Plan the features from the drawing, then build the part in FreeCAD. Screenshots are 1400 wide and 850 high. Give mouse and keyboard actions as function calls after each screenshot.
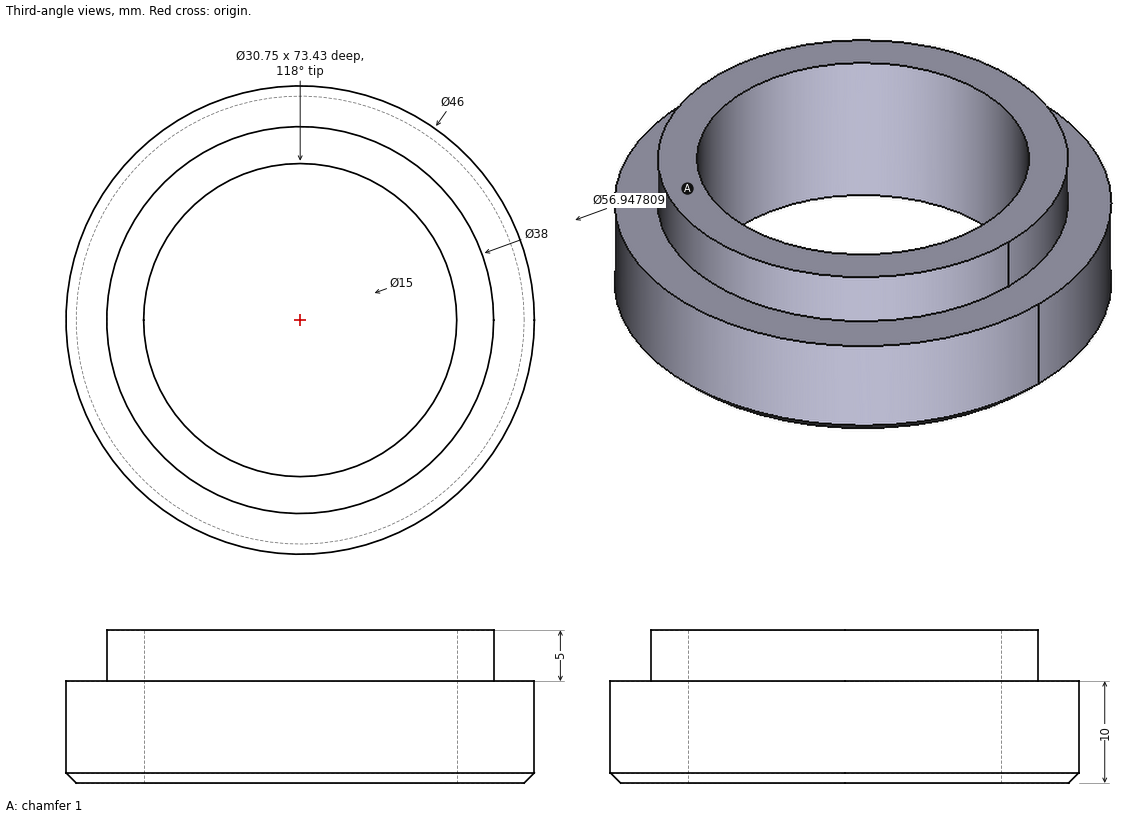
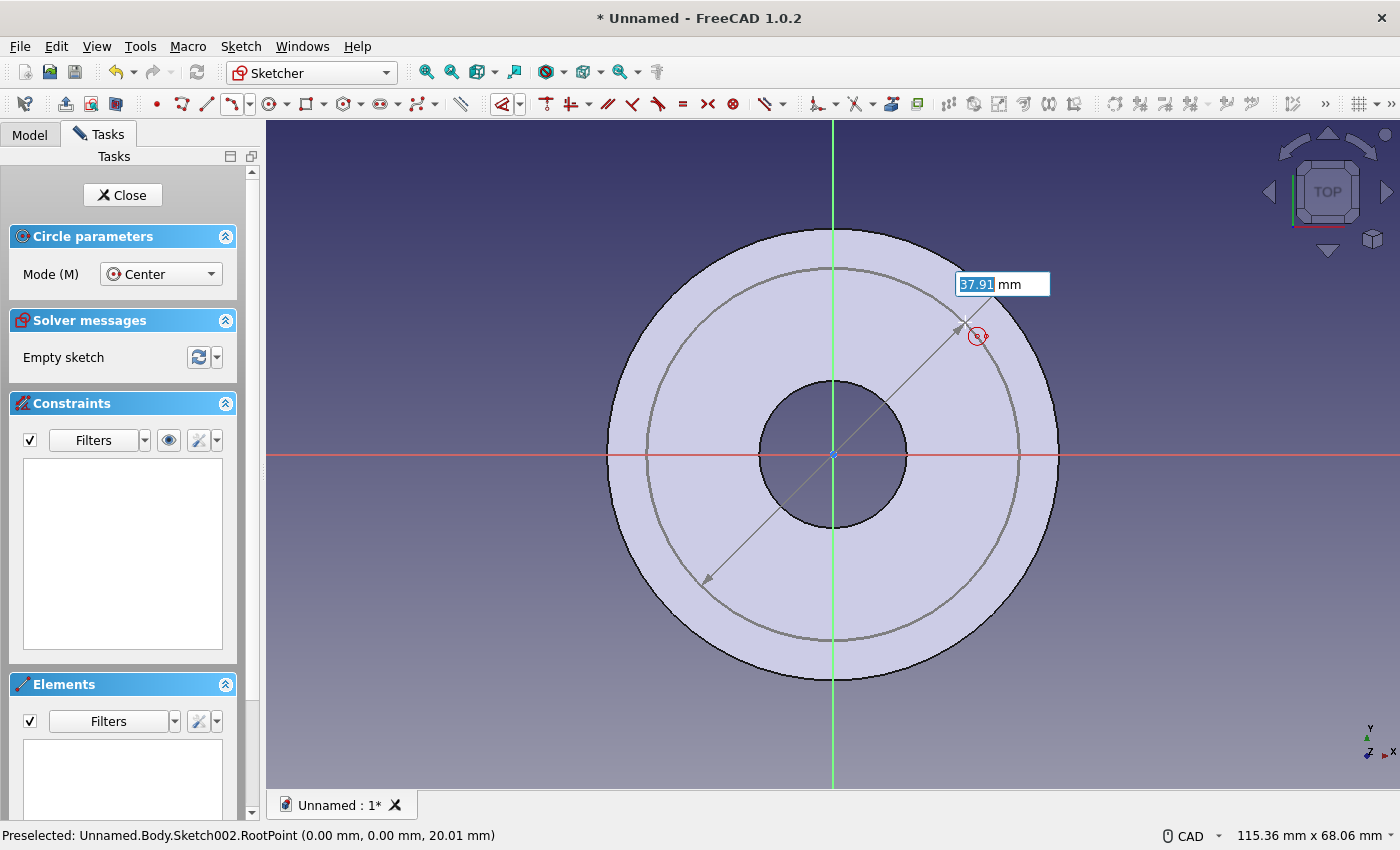
text(38)
key(Return)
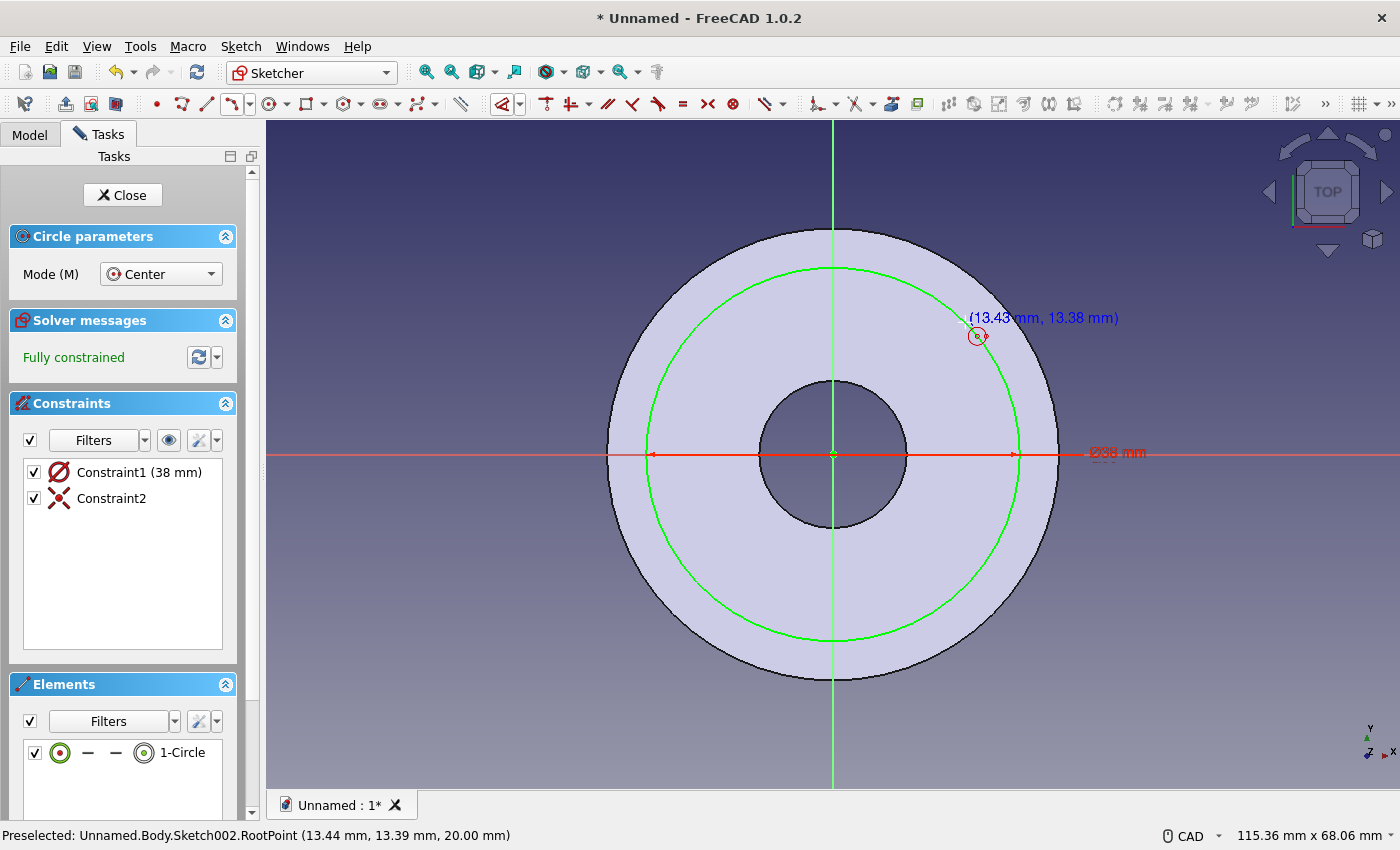
click(833, 454)
move(885, 402)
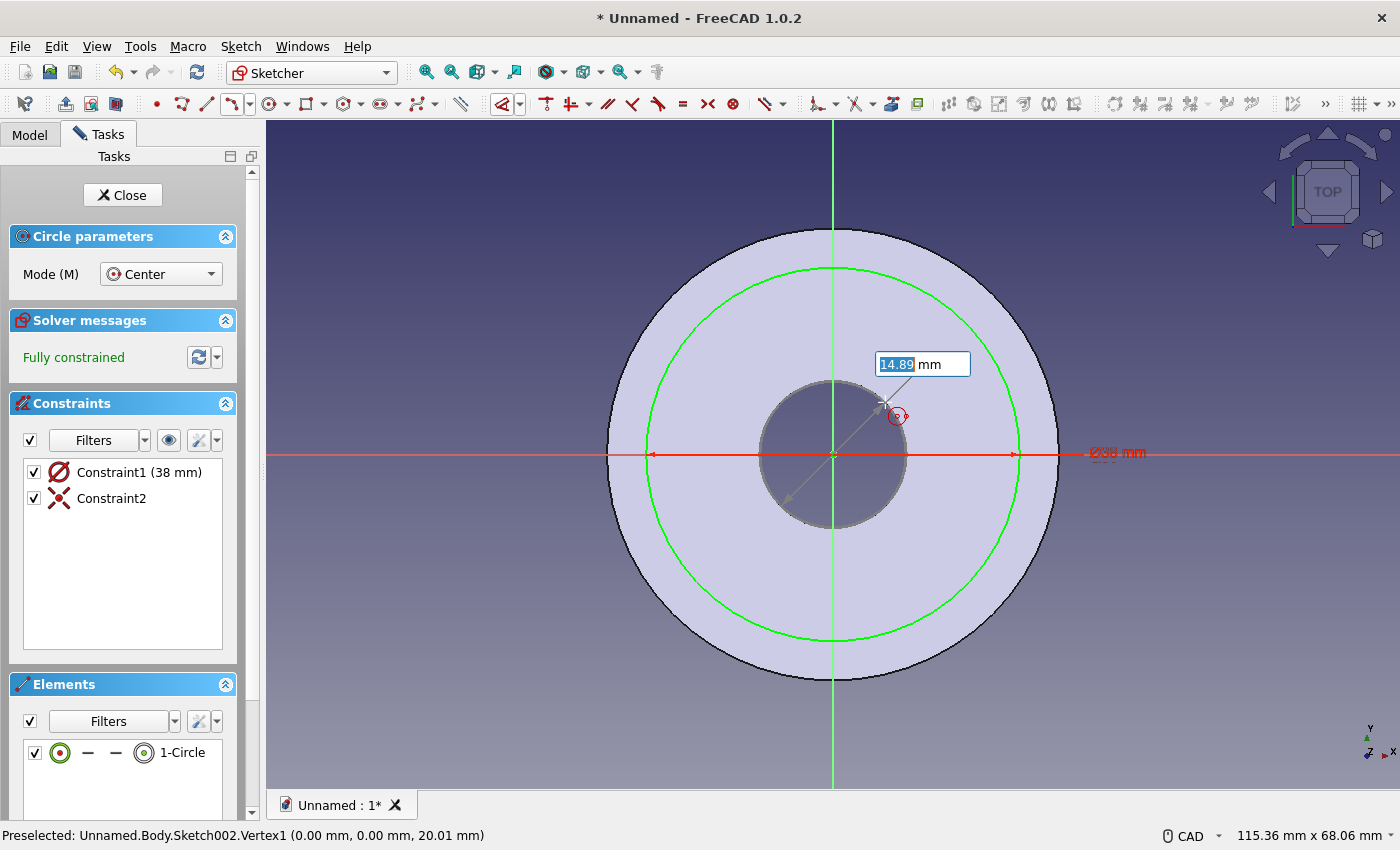
text(15)
key(Return)
key(Escape)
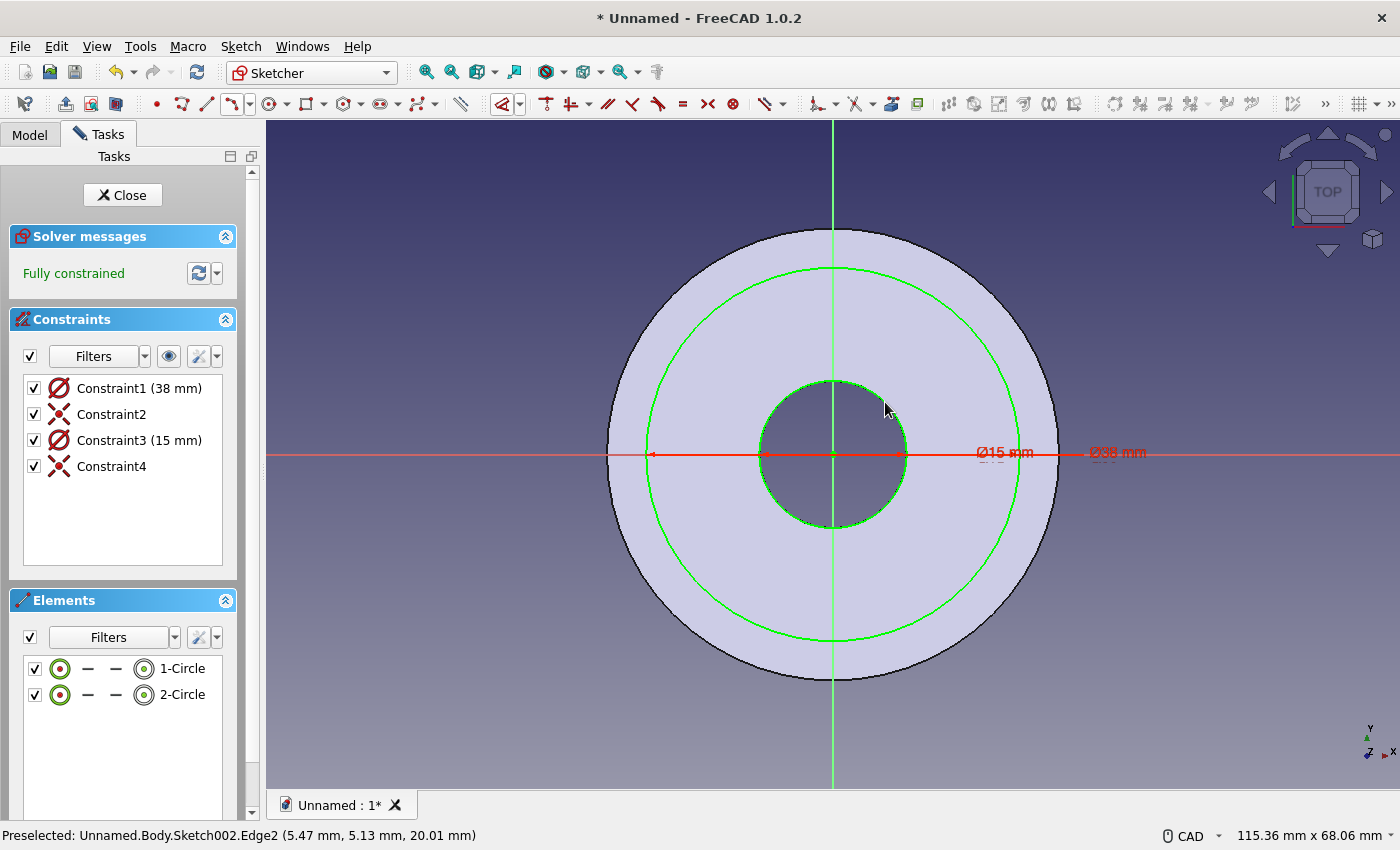
click(123, 195)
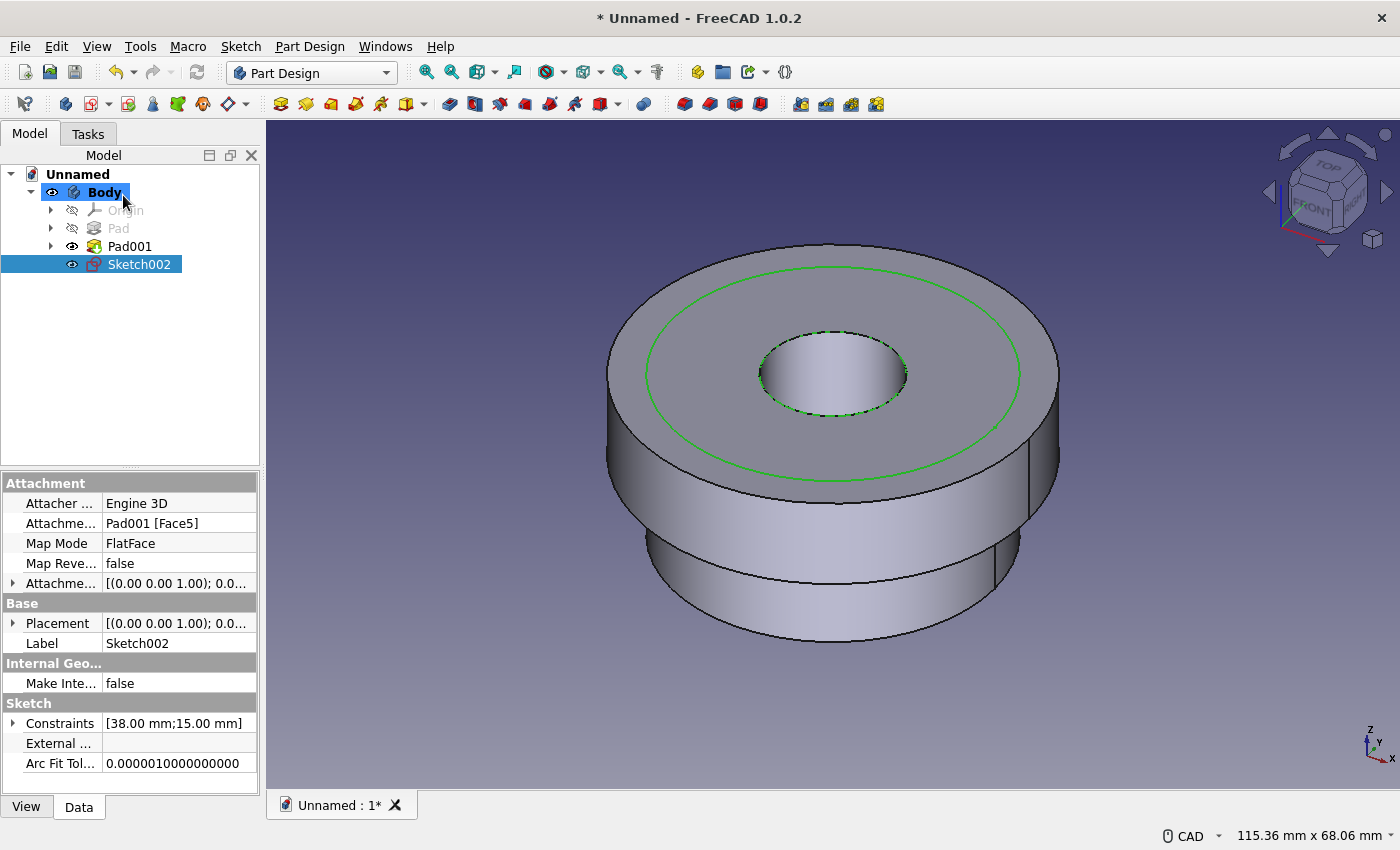
click(281, 104)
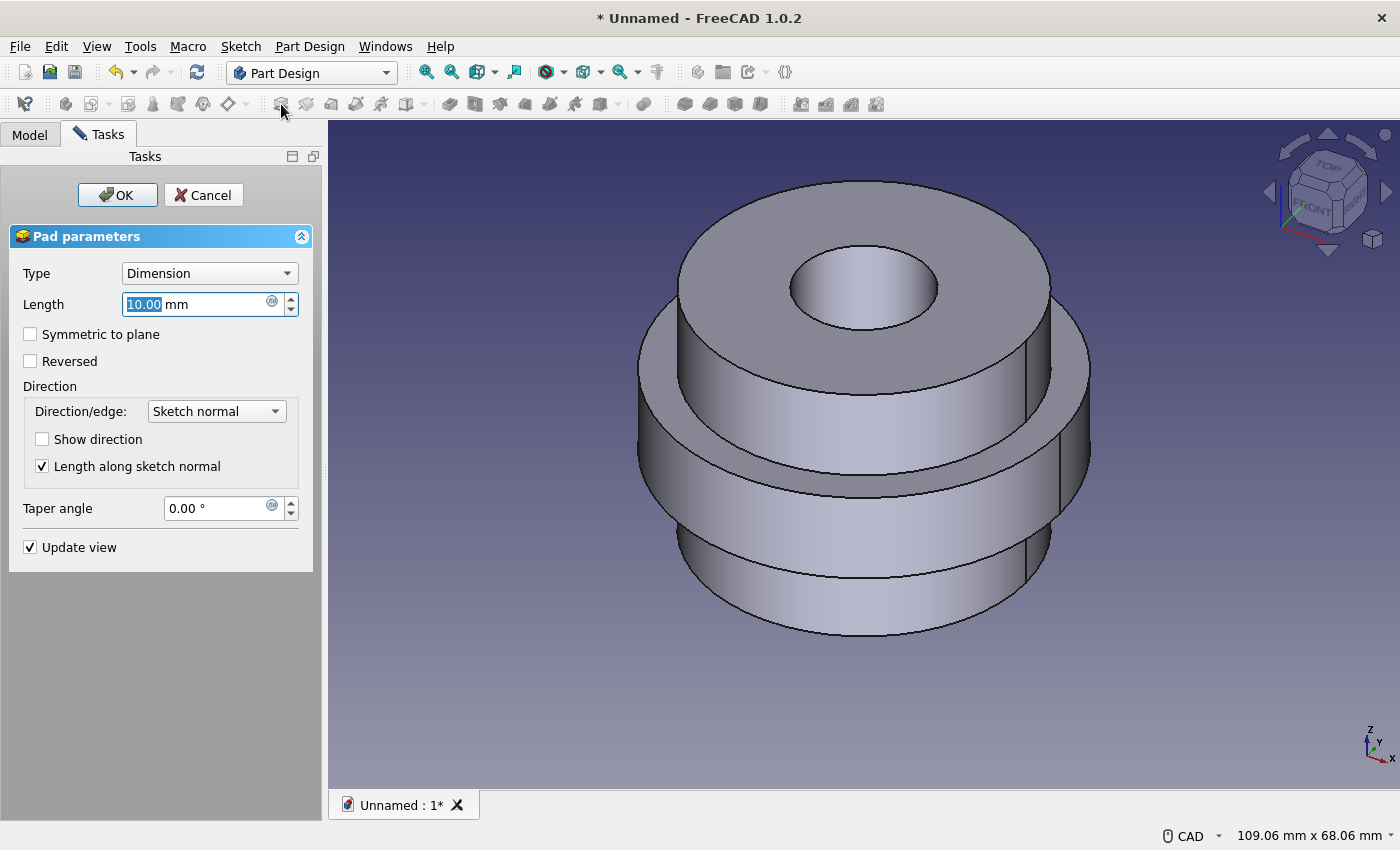
text(5)
key(Tab)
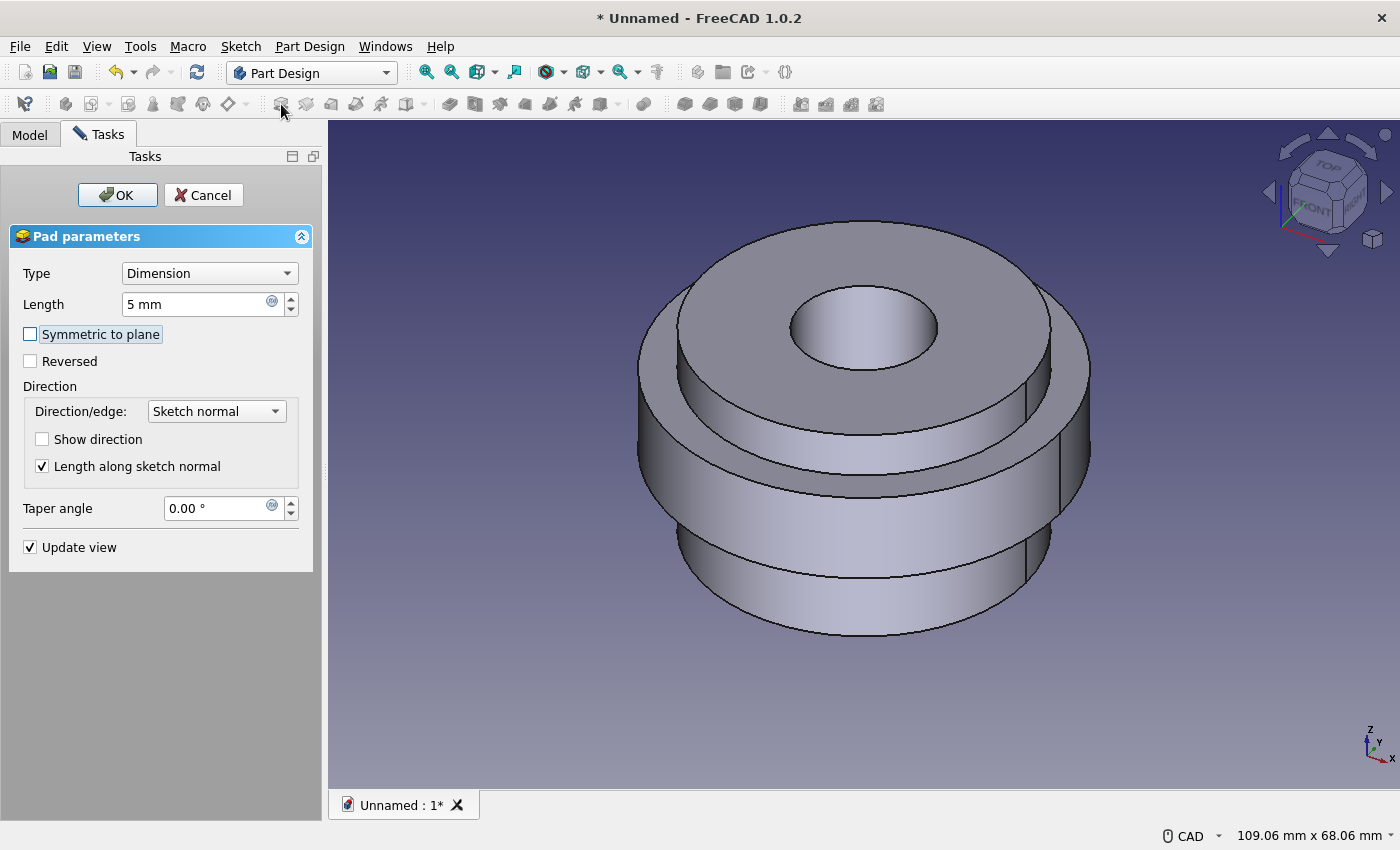
click(118, 195)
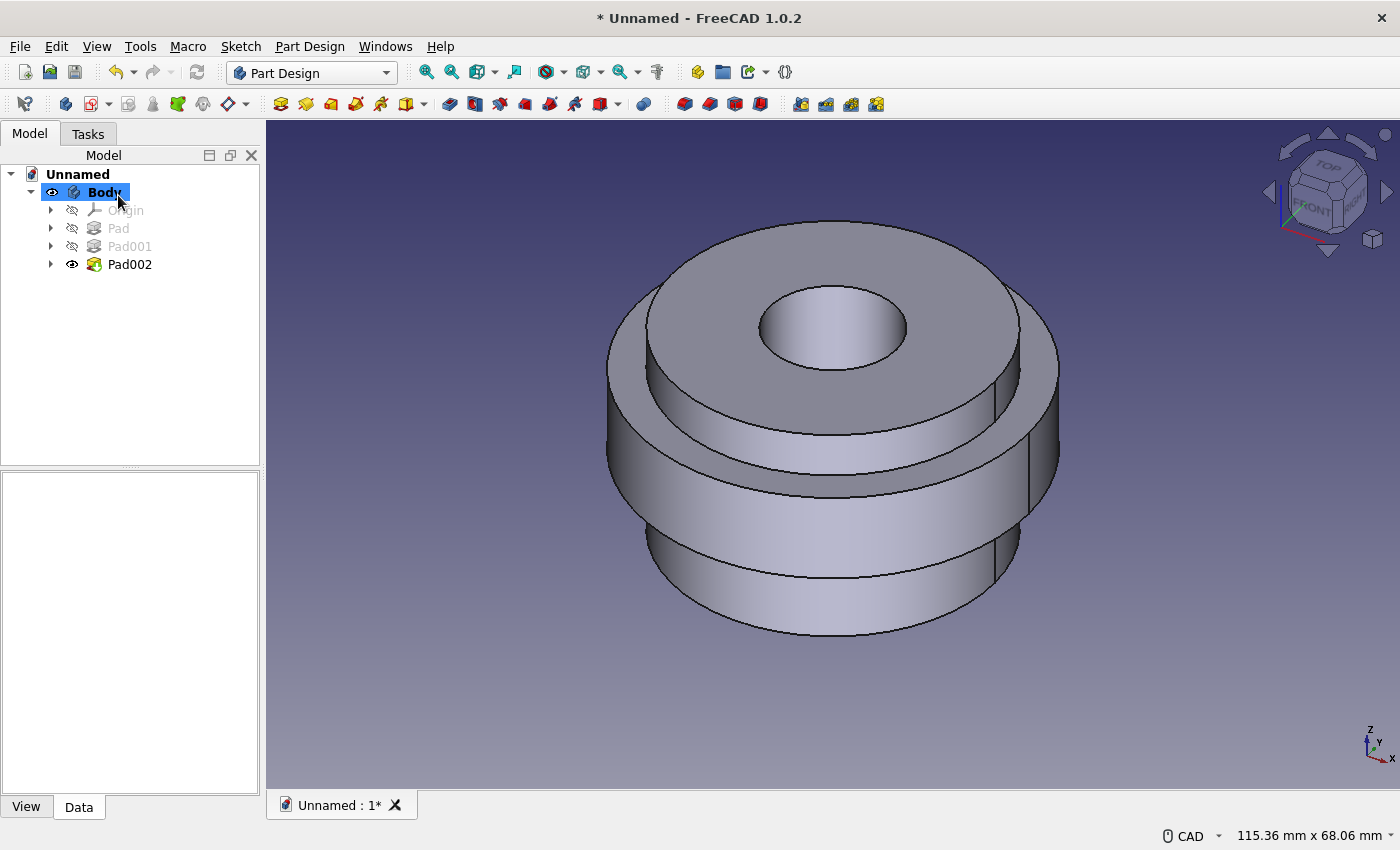
click(840, 259)